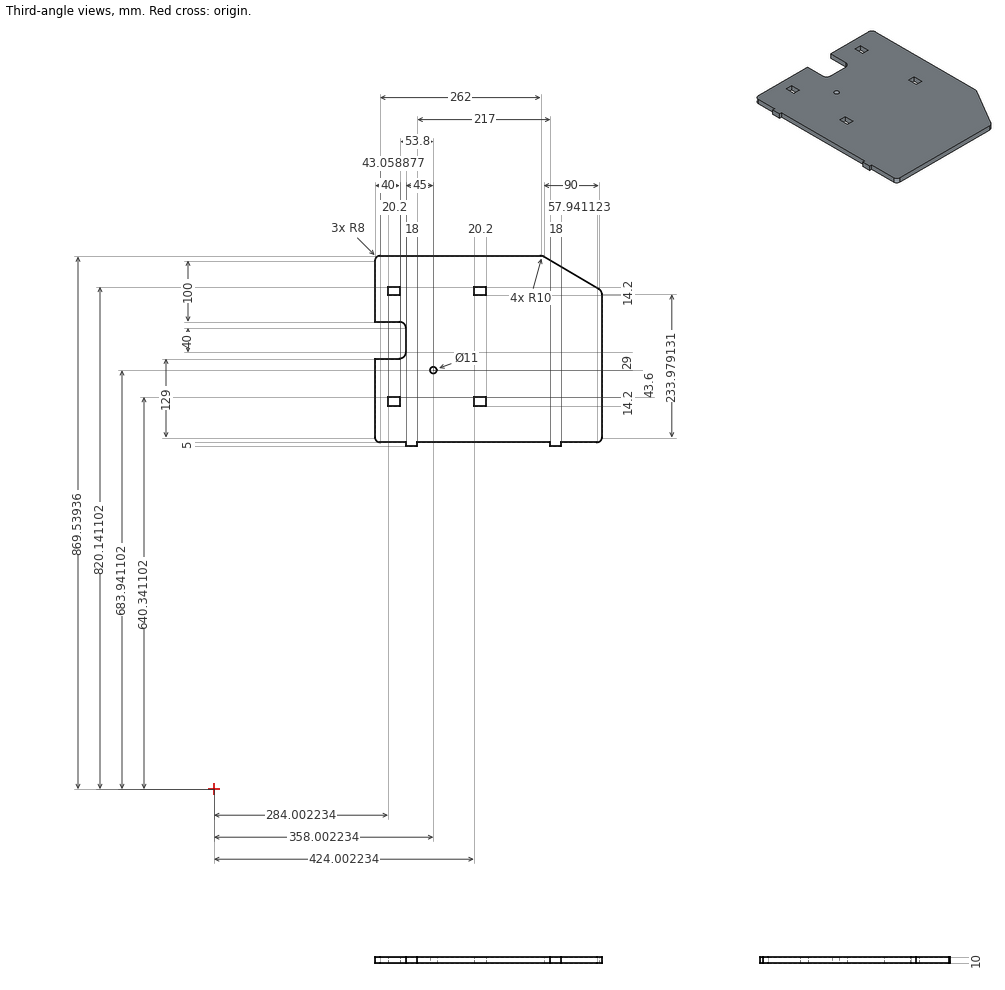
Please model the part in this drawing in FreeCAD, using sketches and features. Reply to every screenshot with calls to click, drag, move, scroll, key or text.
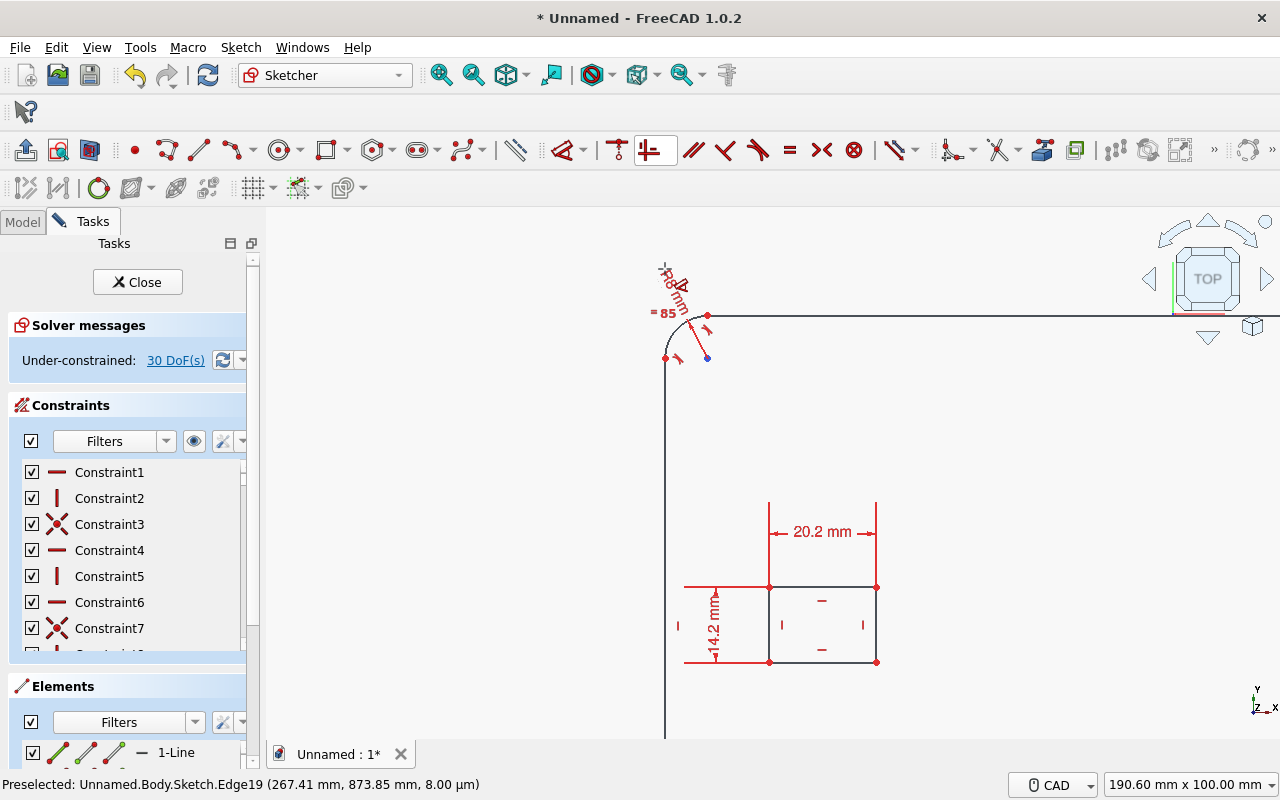
scroll(685, 300, down, 13)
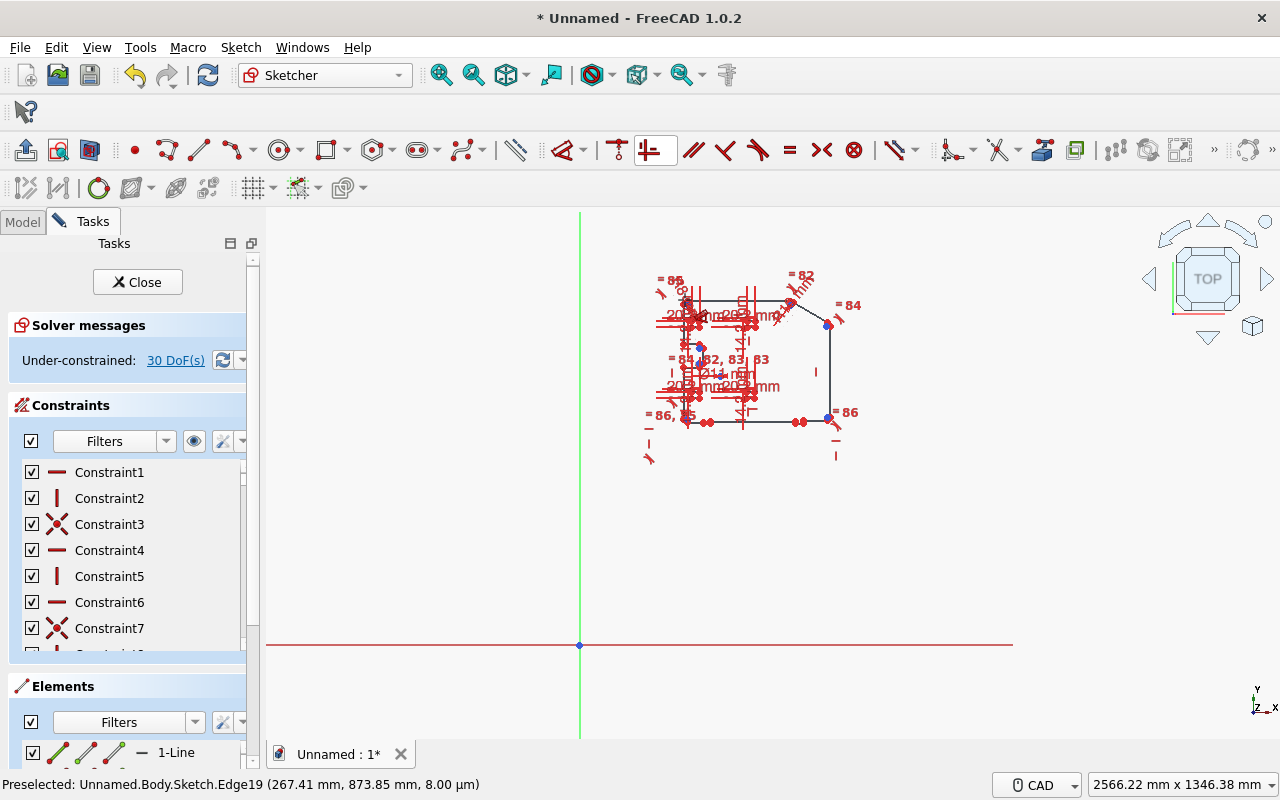
scroll(704, 423, up, 16)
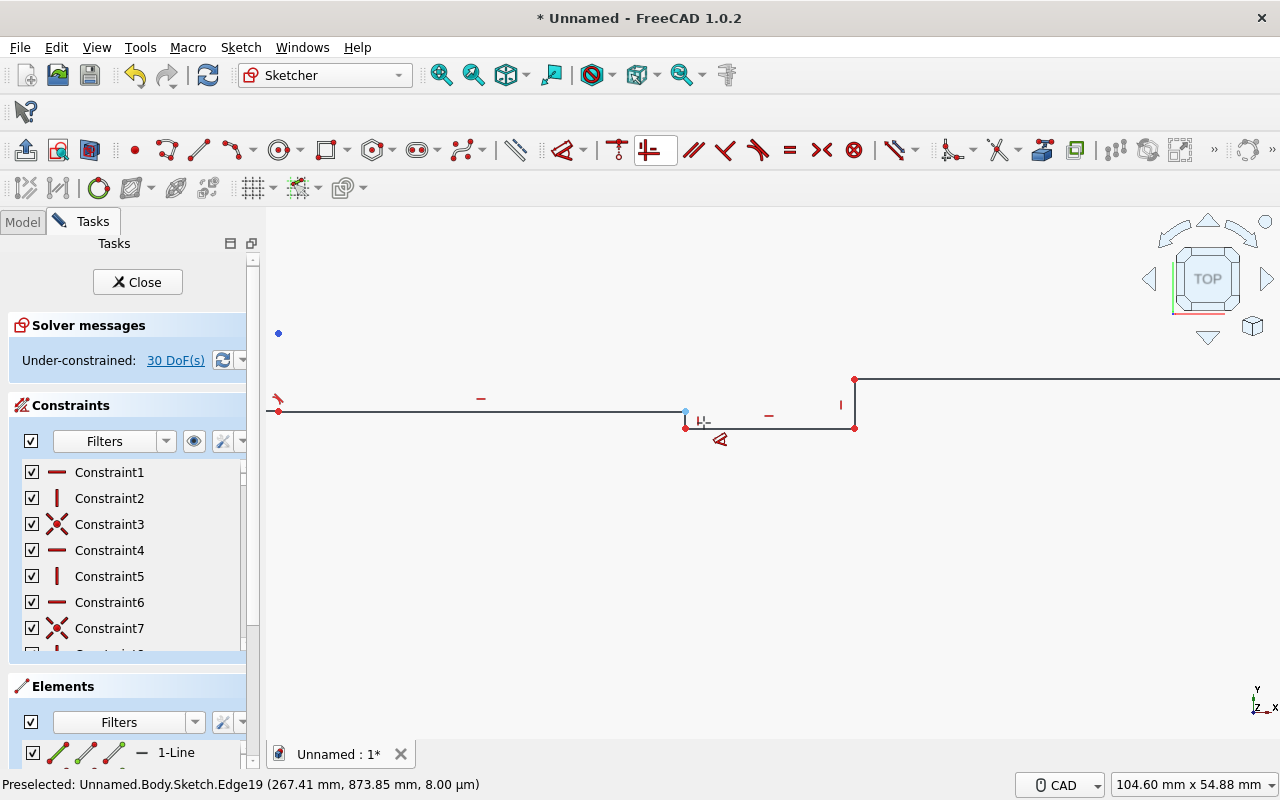
click(685, 420)
click(651, 426)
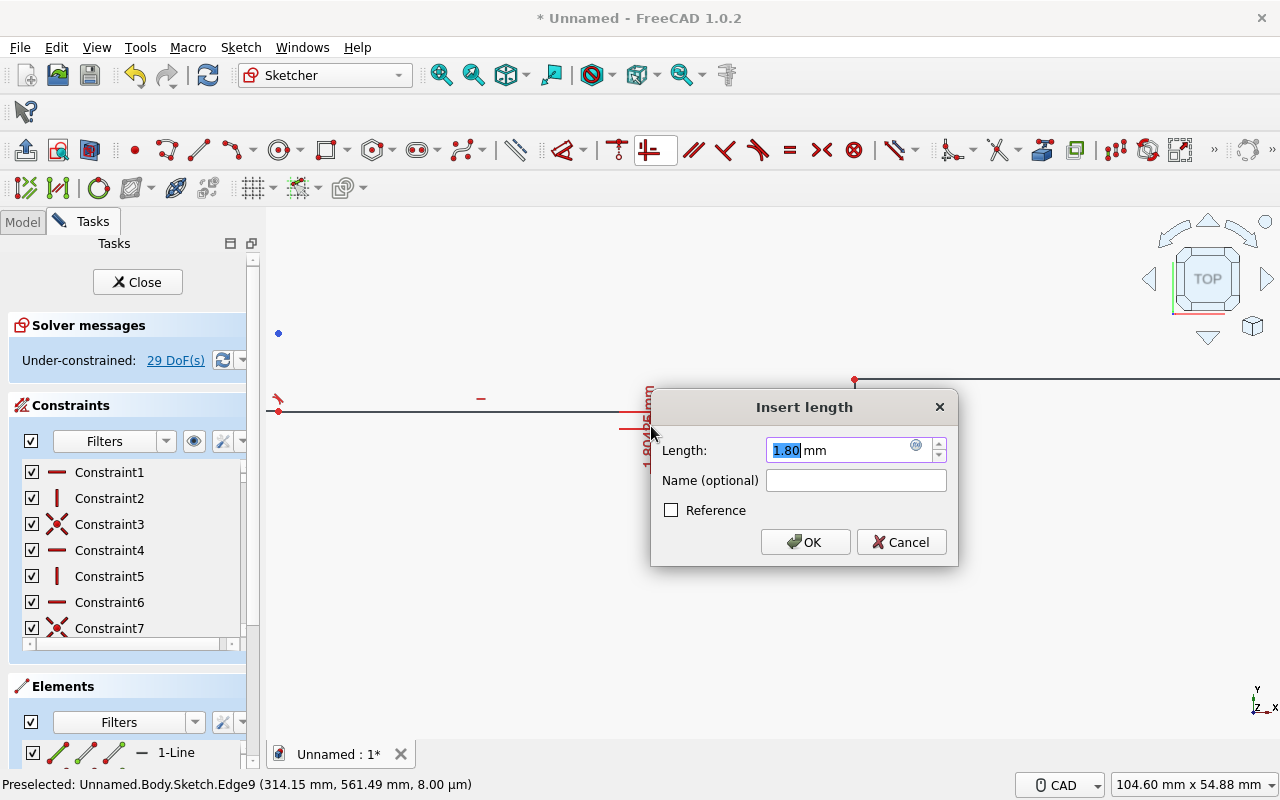
text(5)
key(Return)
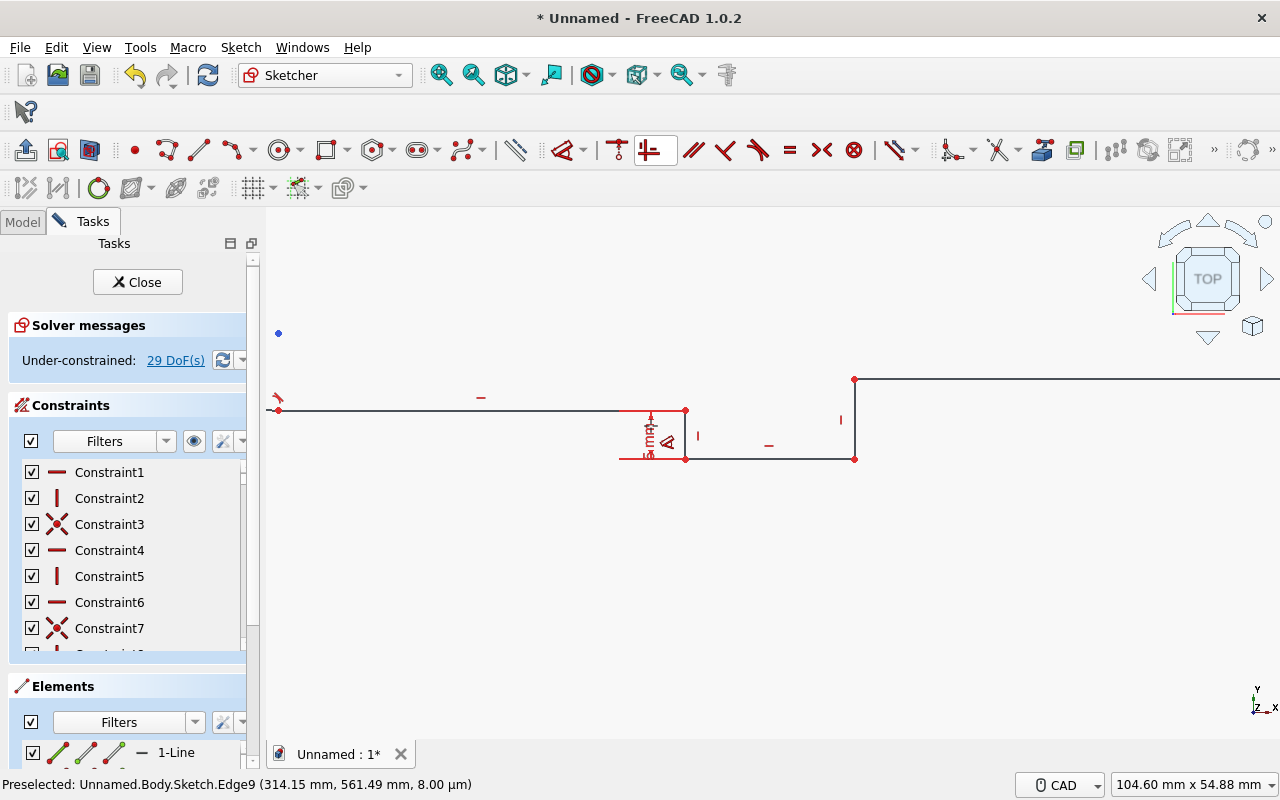
click(855, 435)
click(889, 419)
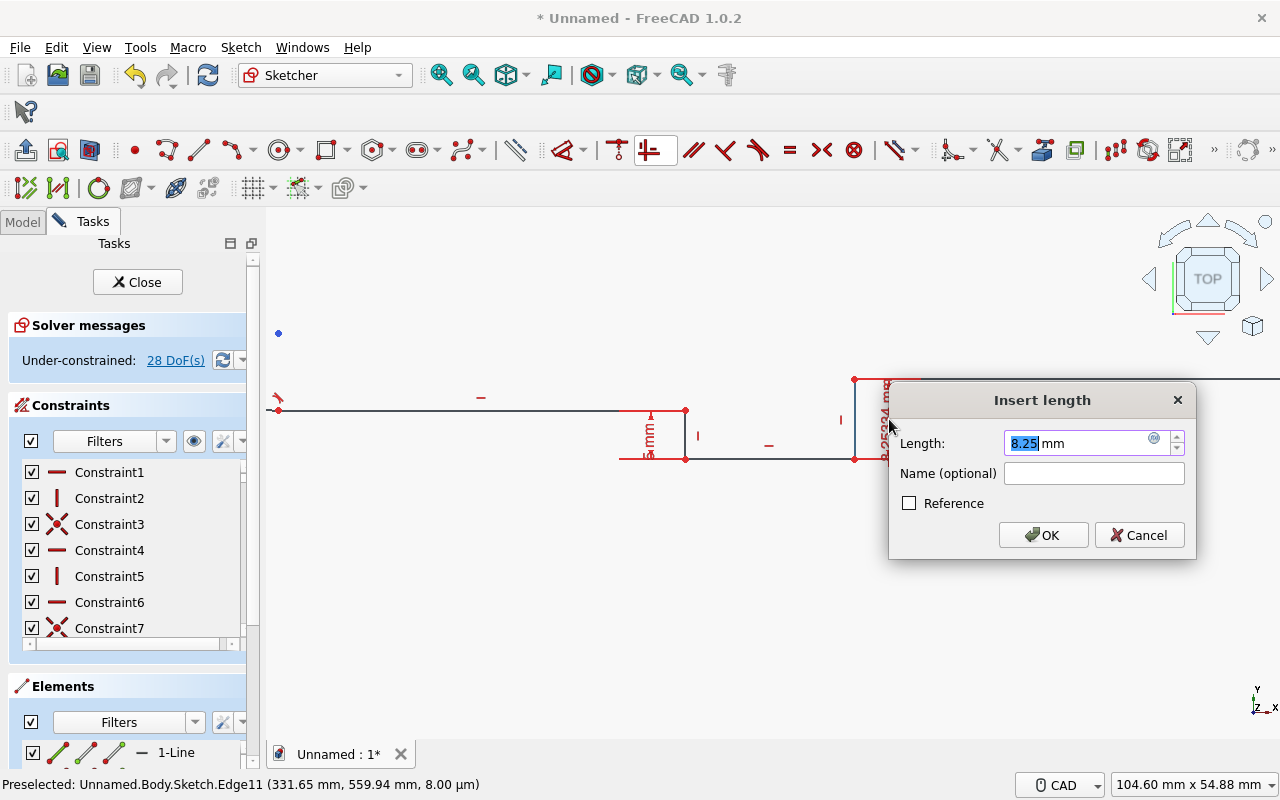
text(5)
key(Return)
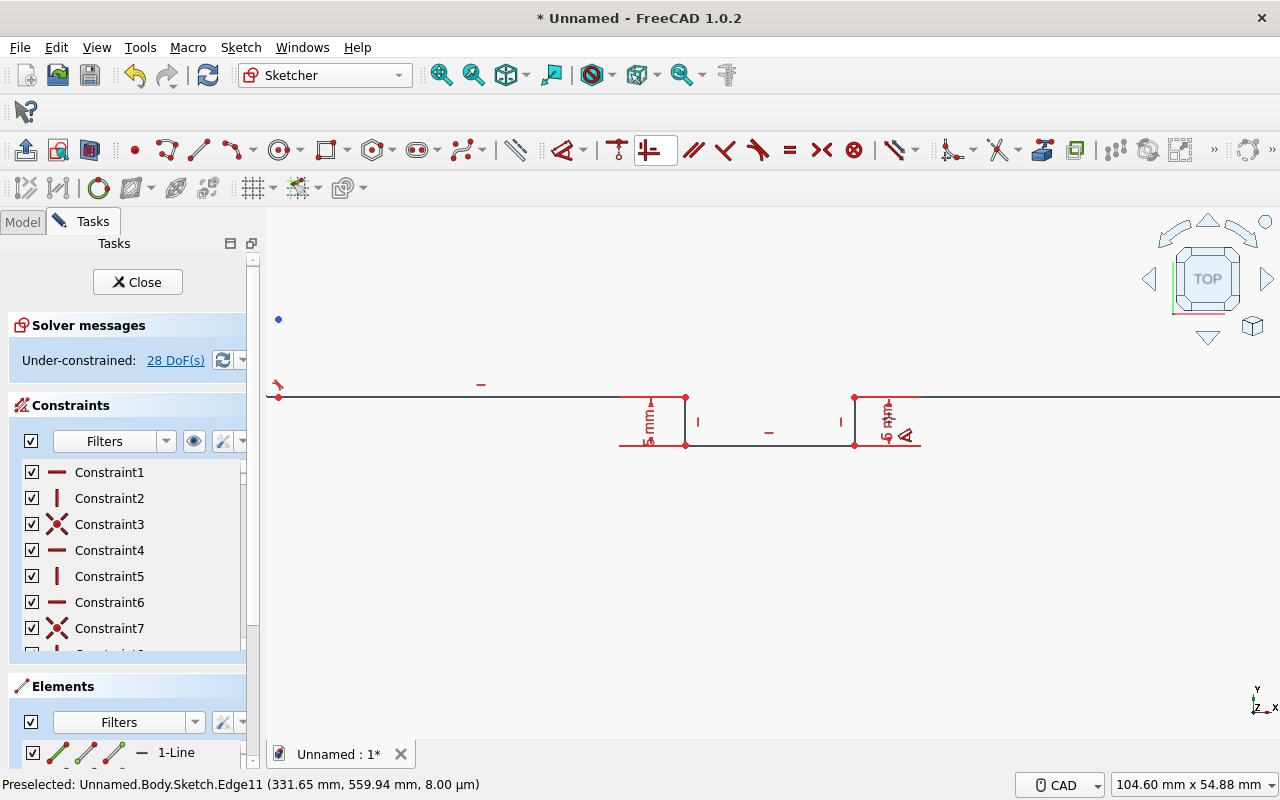
scroll(704, 412, down, 15)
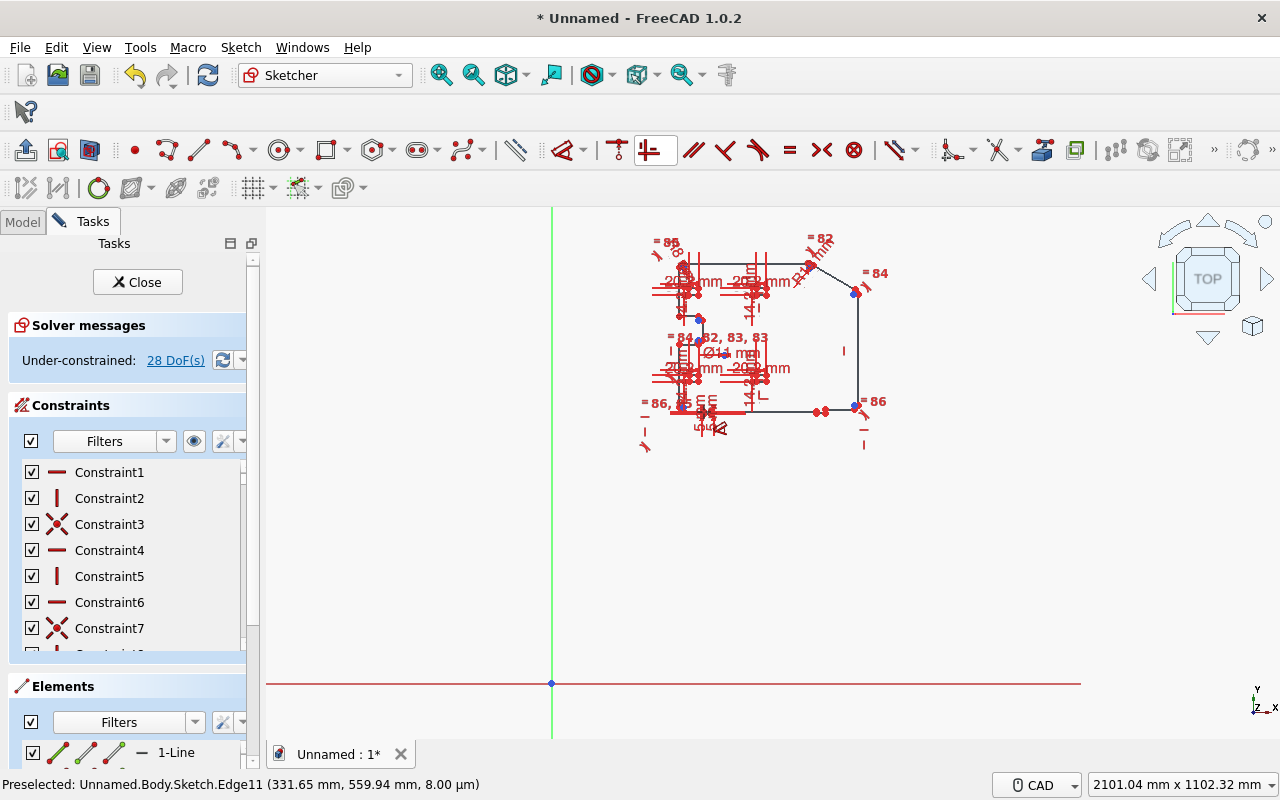
scroll(816, 412, up, 15)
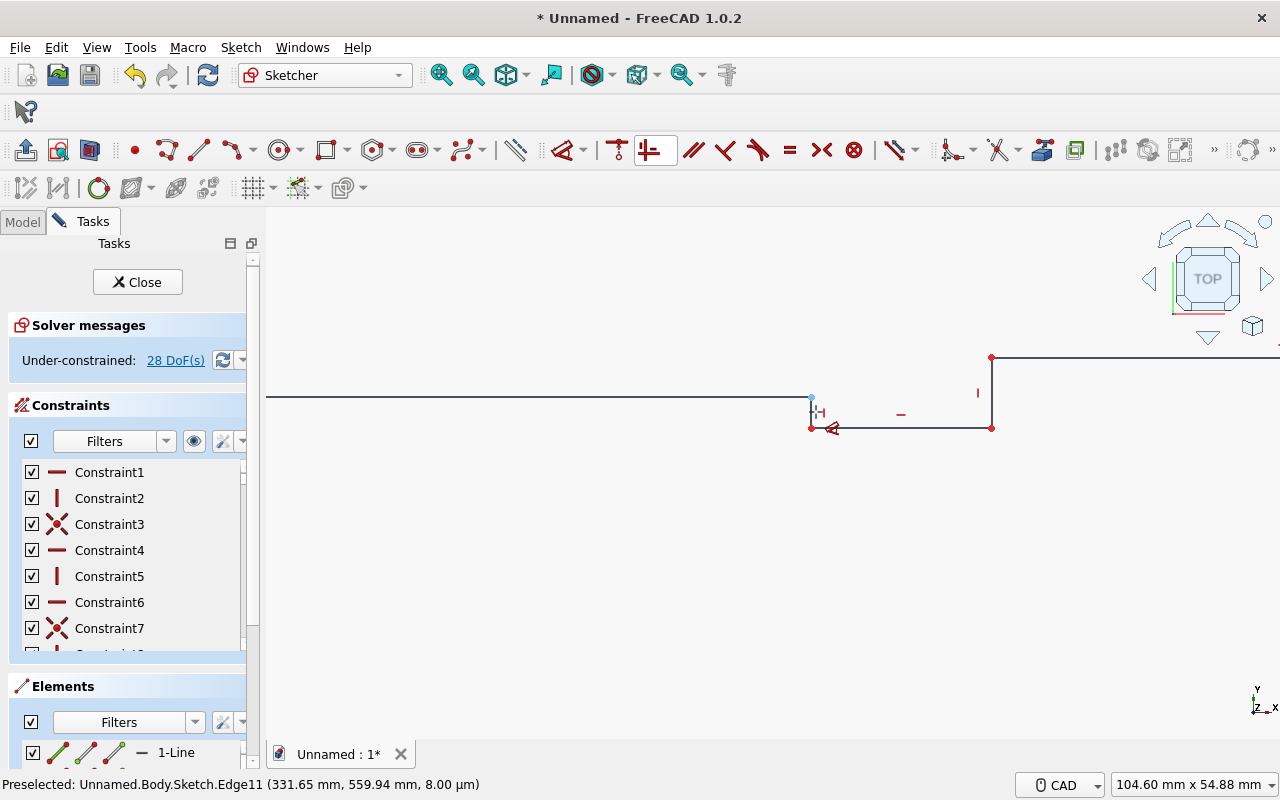
click(811, 407)
click(845, 413)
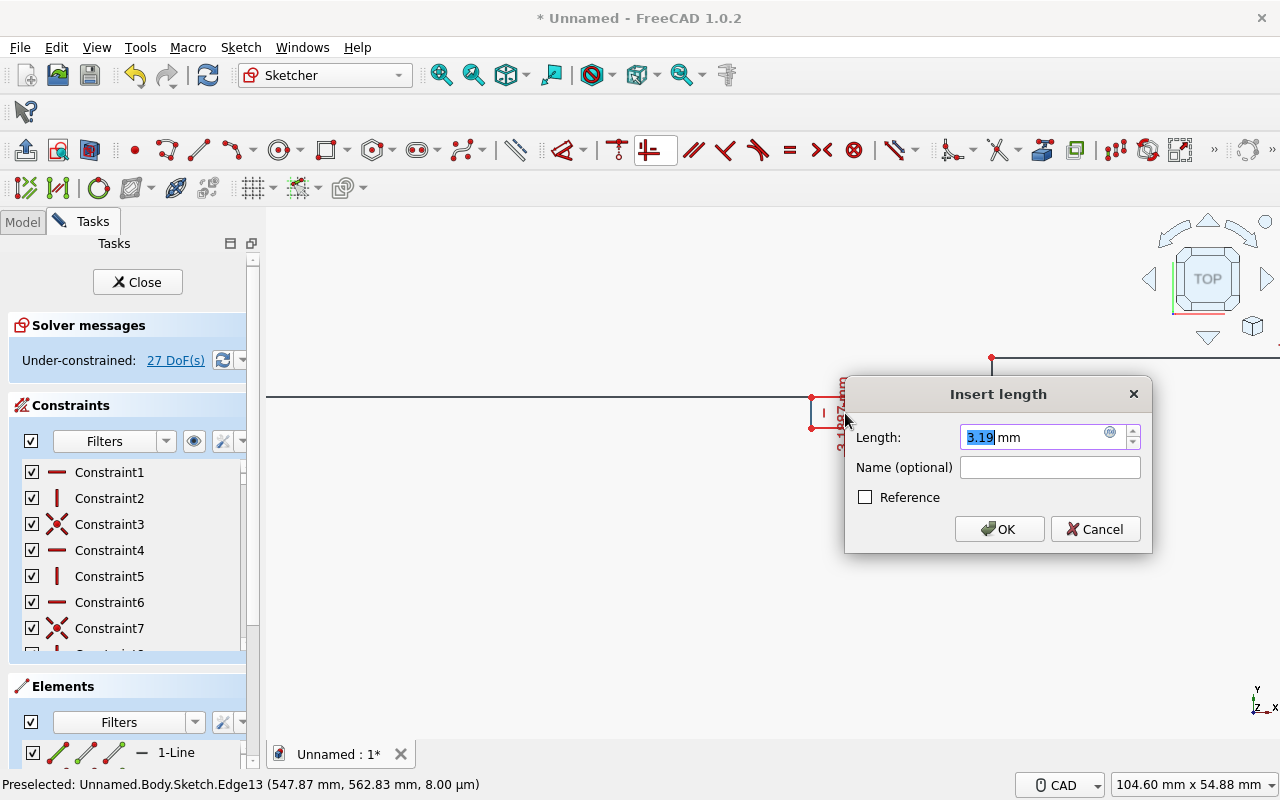
text(5)
key(Return)